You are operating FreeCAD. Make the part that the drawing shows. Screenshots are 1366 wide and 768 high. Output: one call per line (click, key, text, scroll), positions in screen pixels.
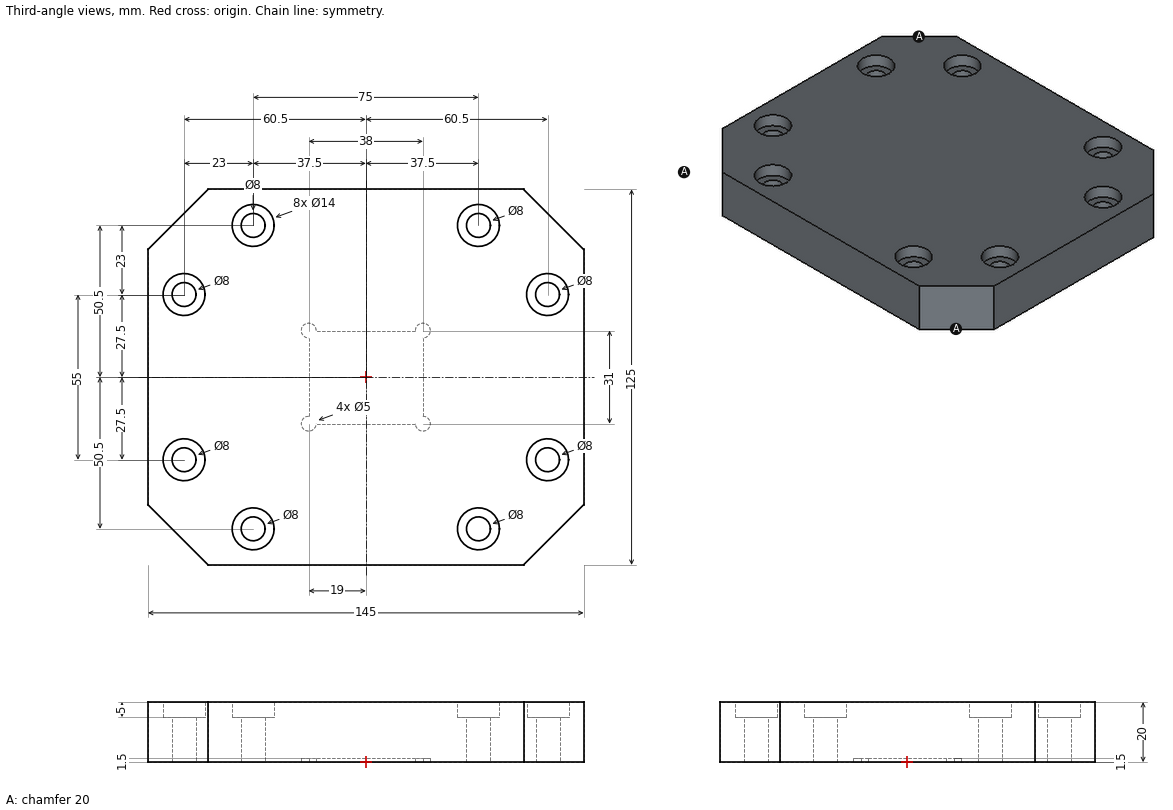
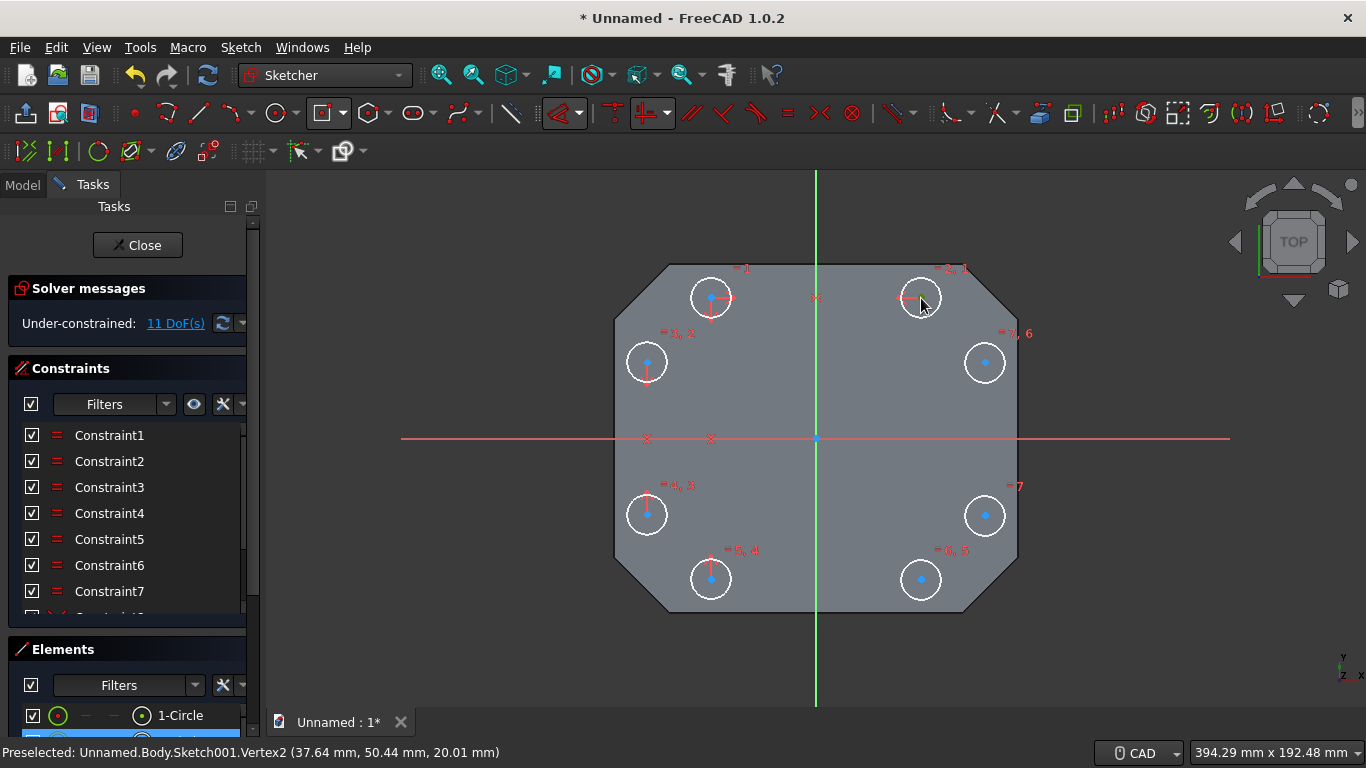
click(921, 580)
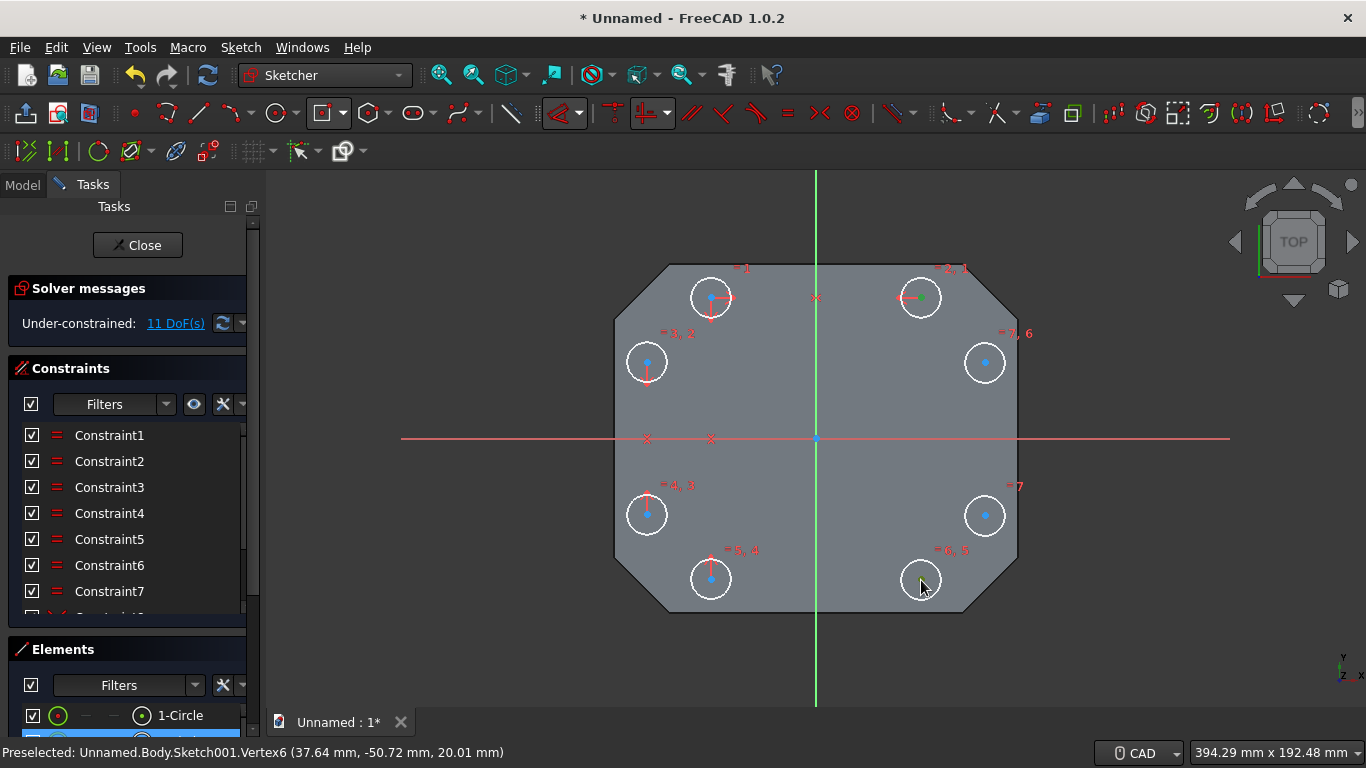
click(424, 438)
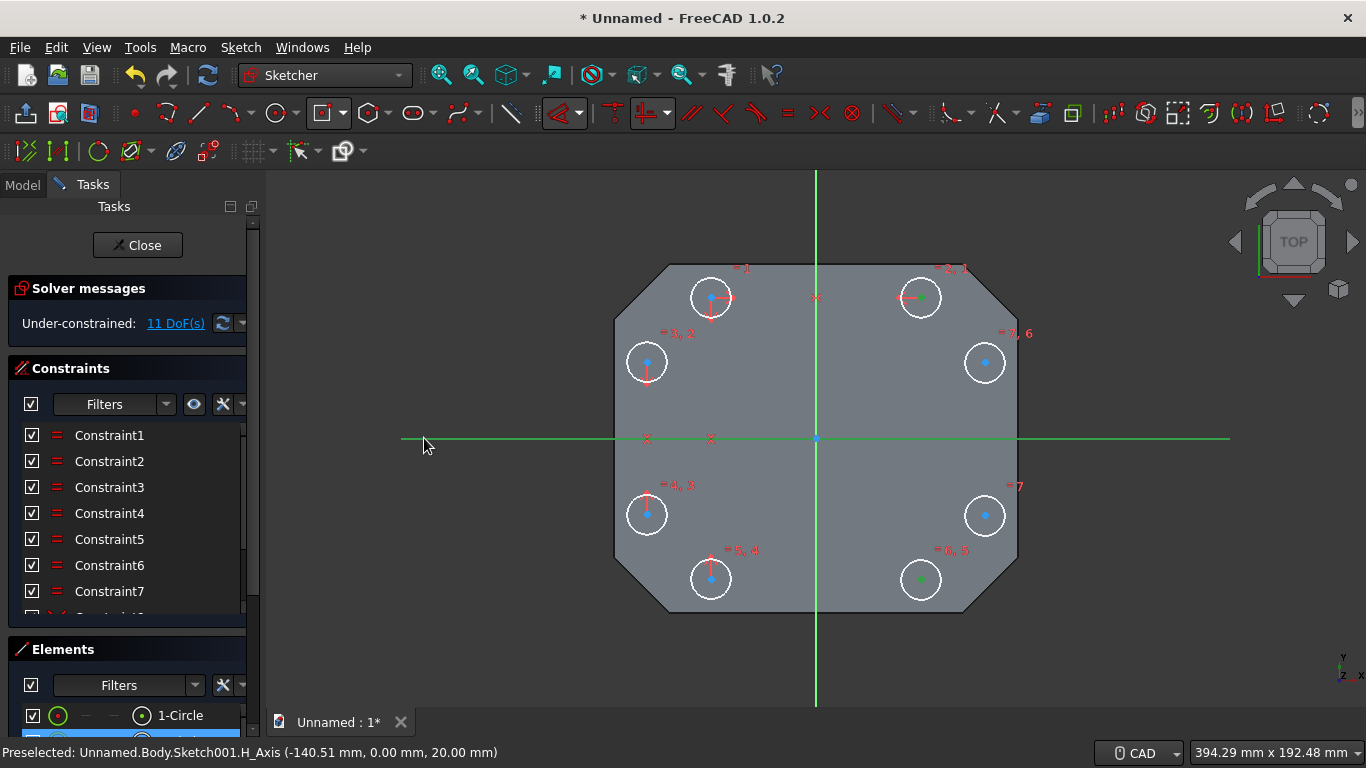
key(s)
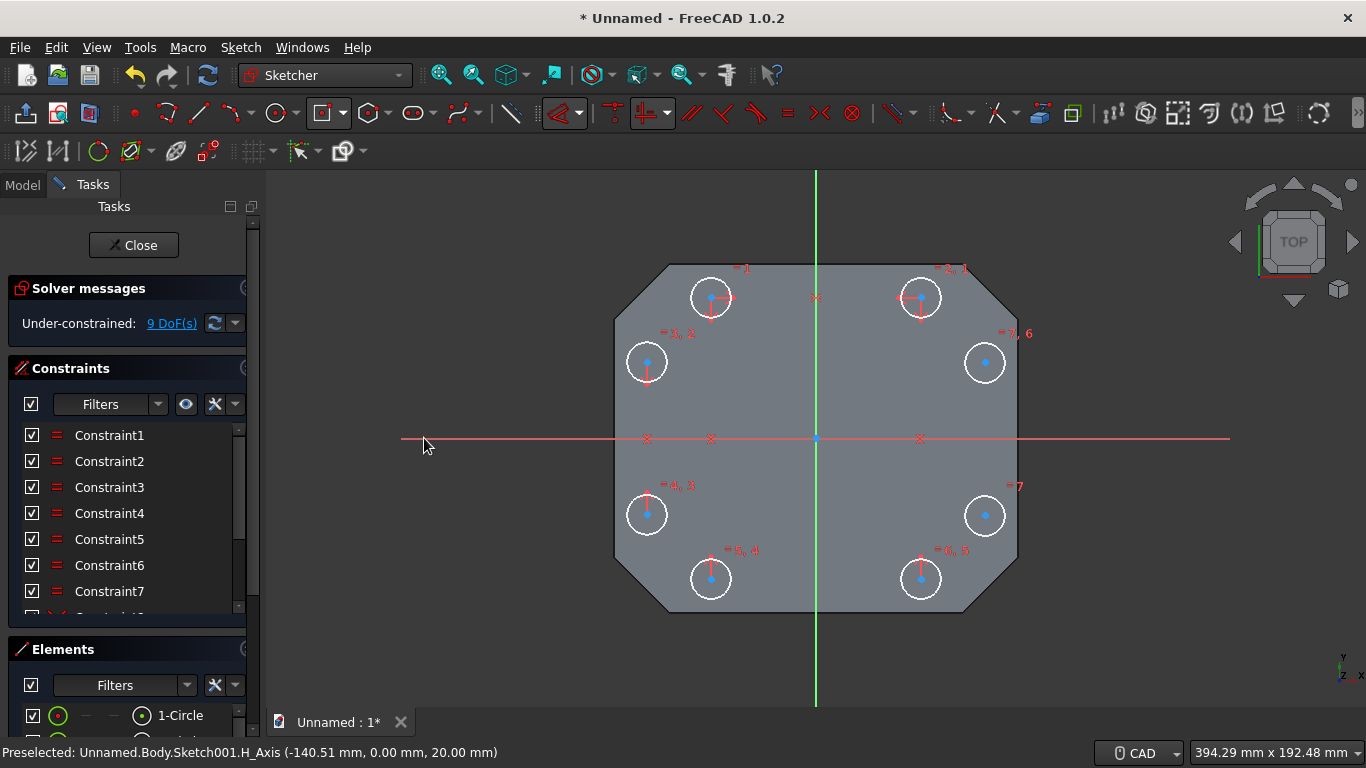
click(647, 362)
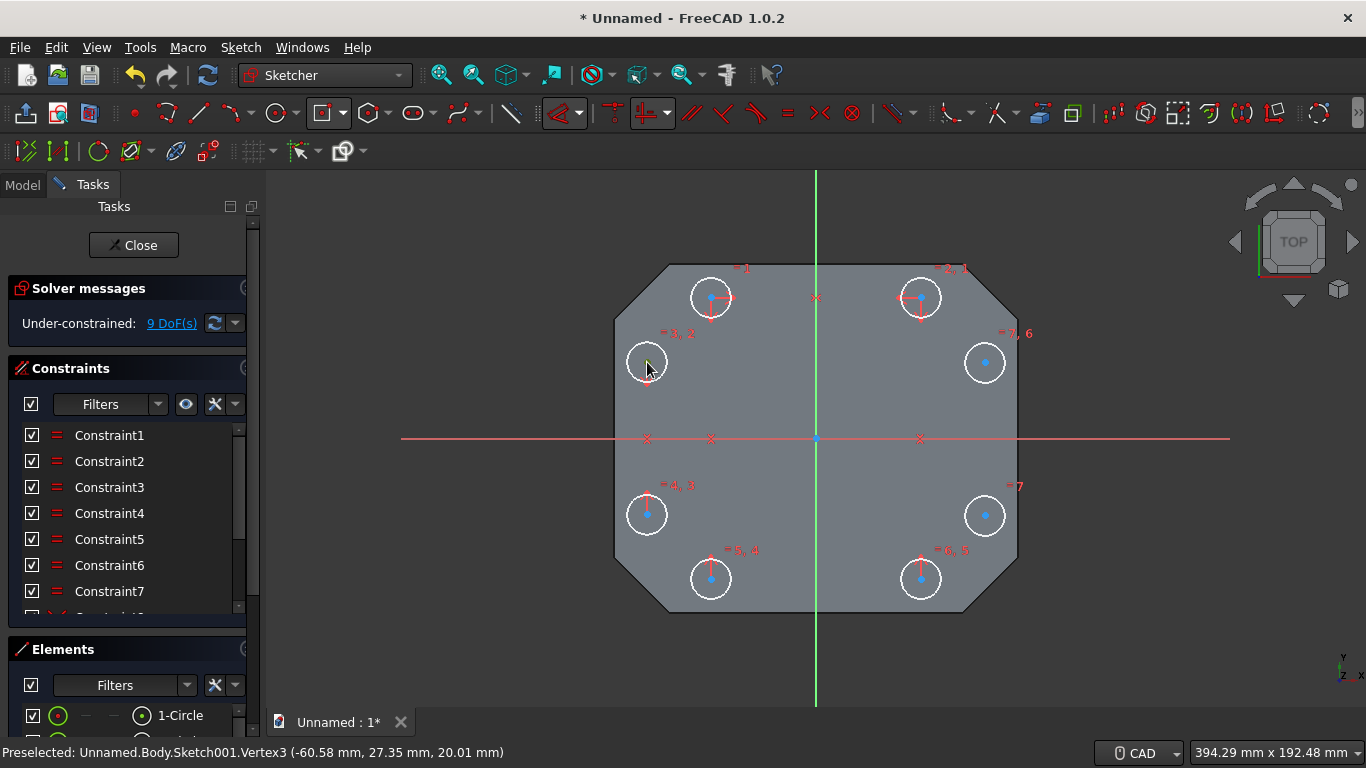
click(985, 363)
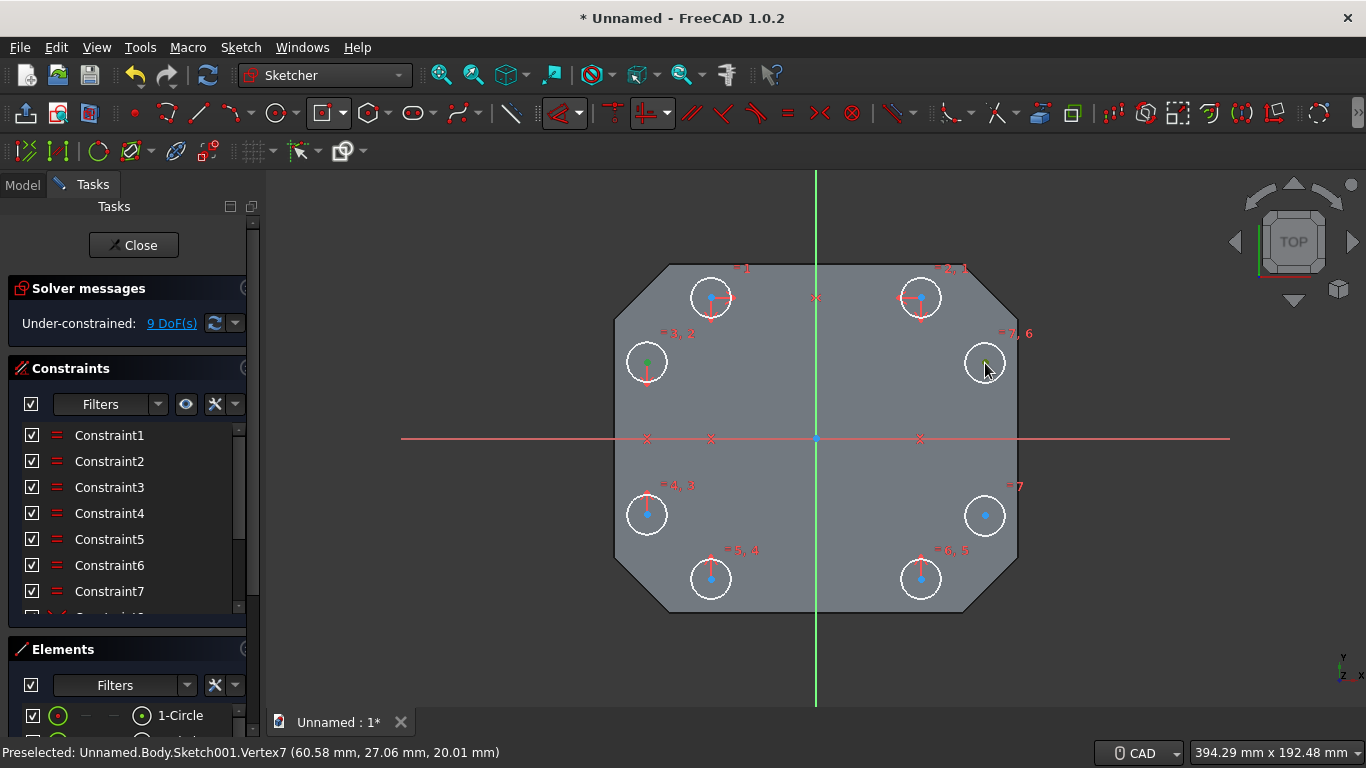
click(816, 645)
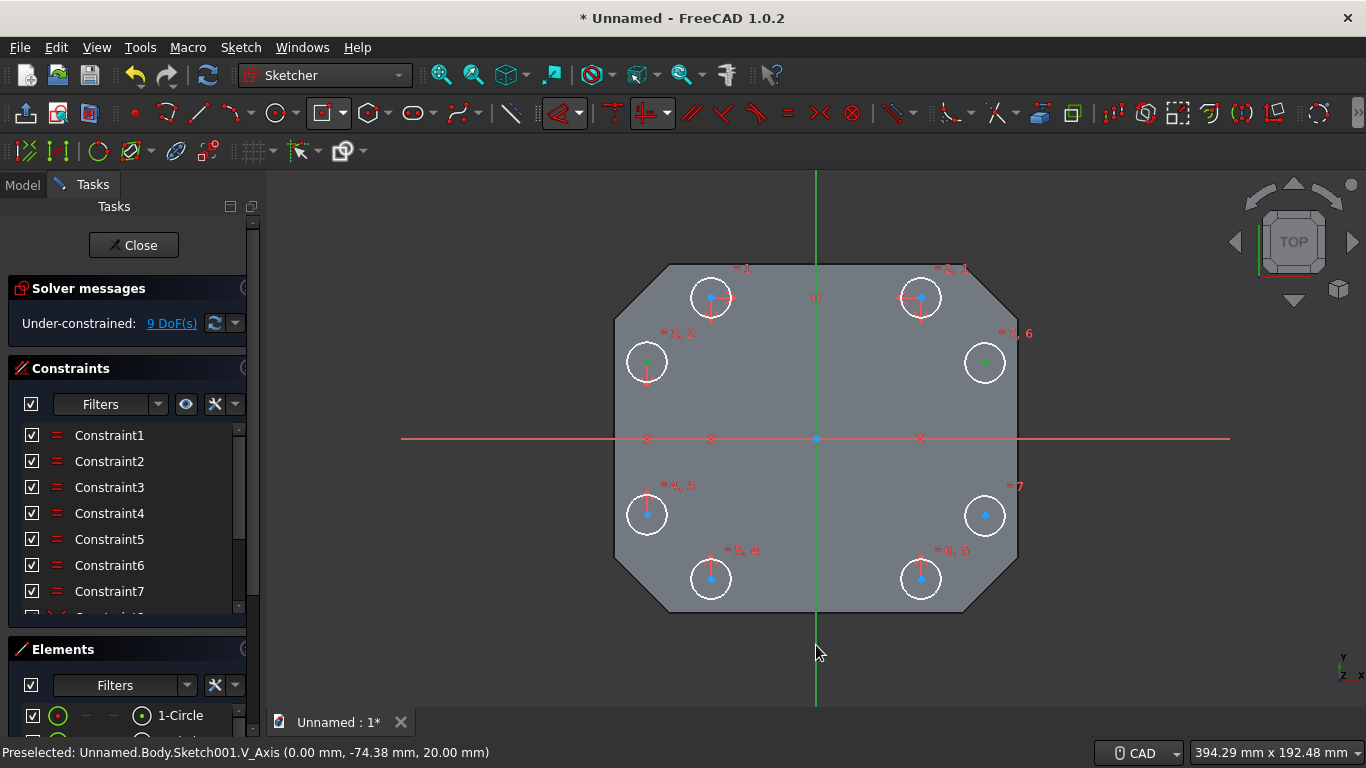
click(820, 114)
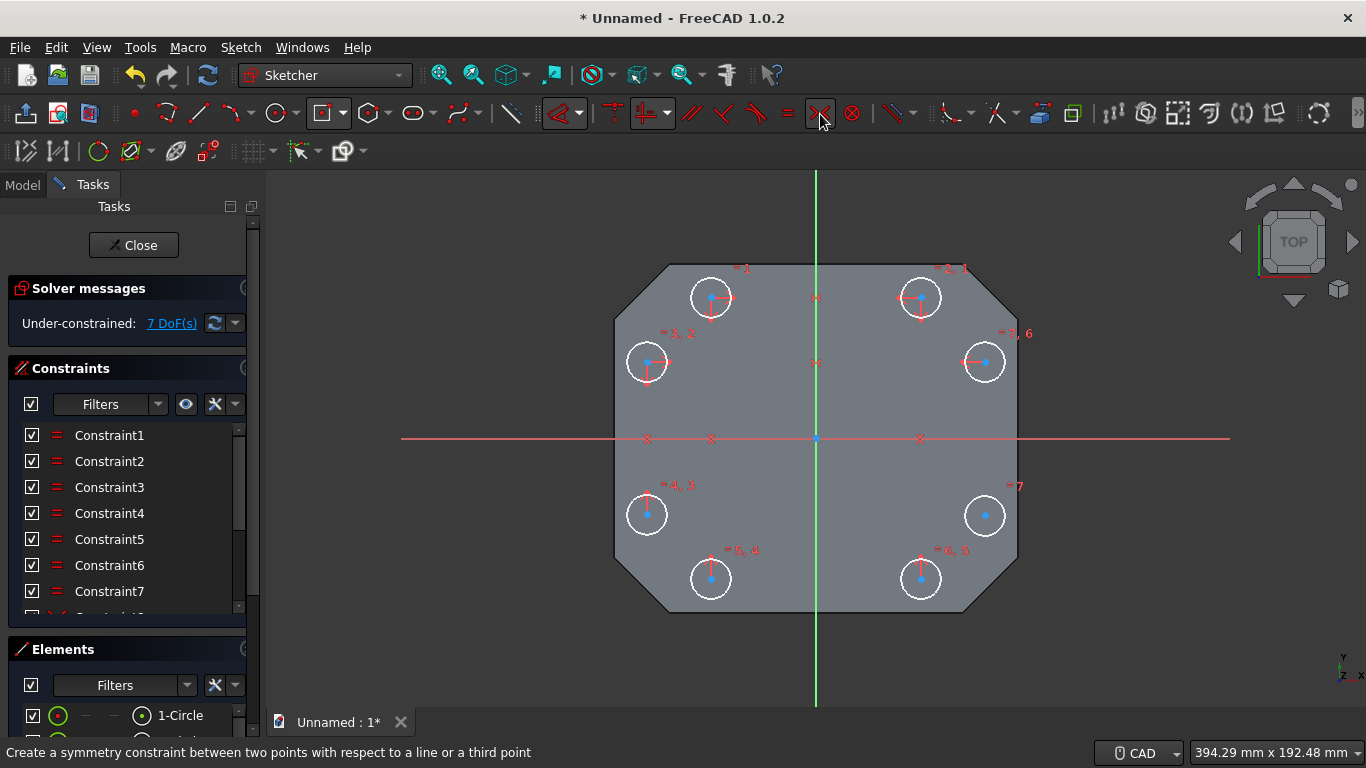
click(647, 515)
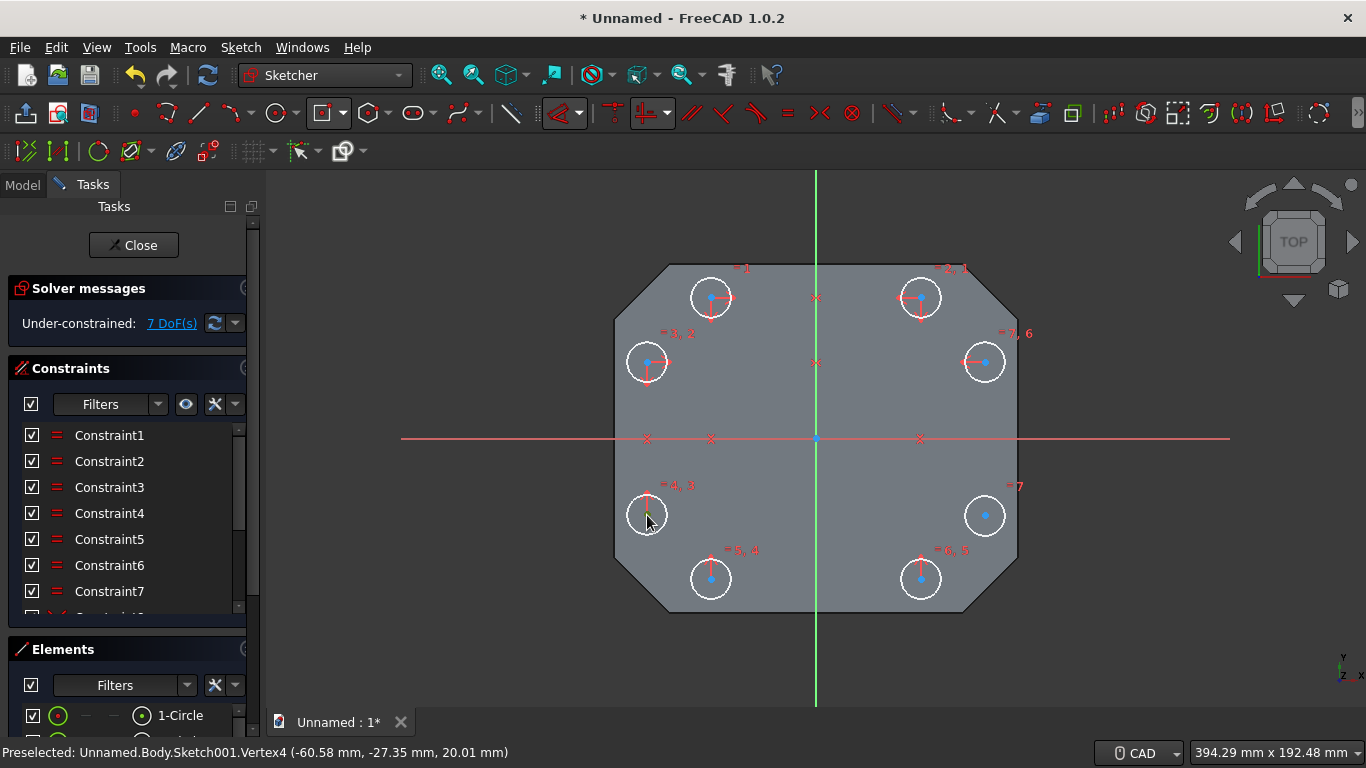
click(985, 516)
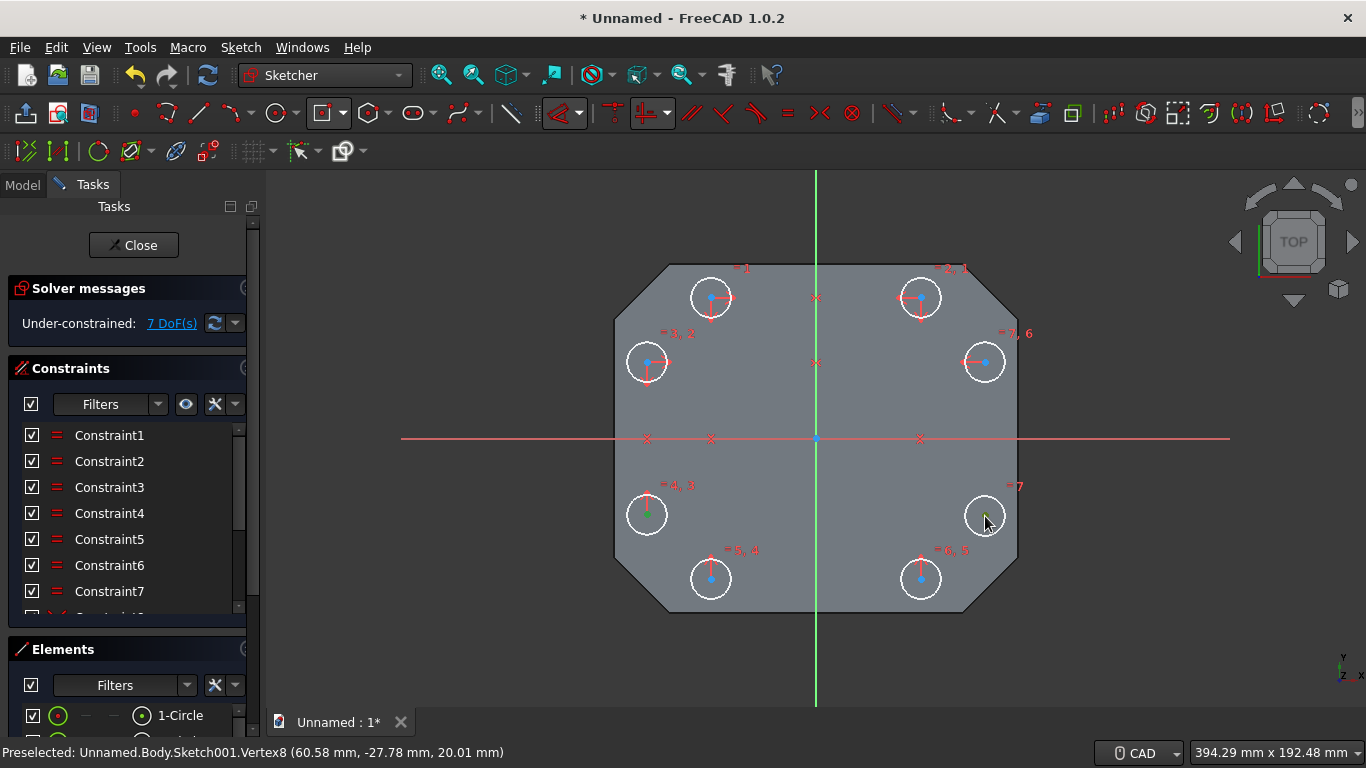
click(816, 645)